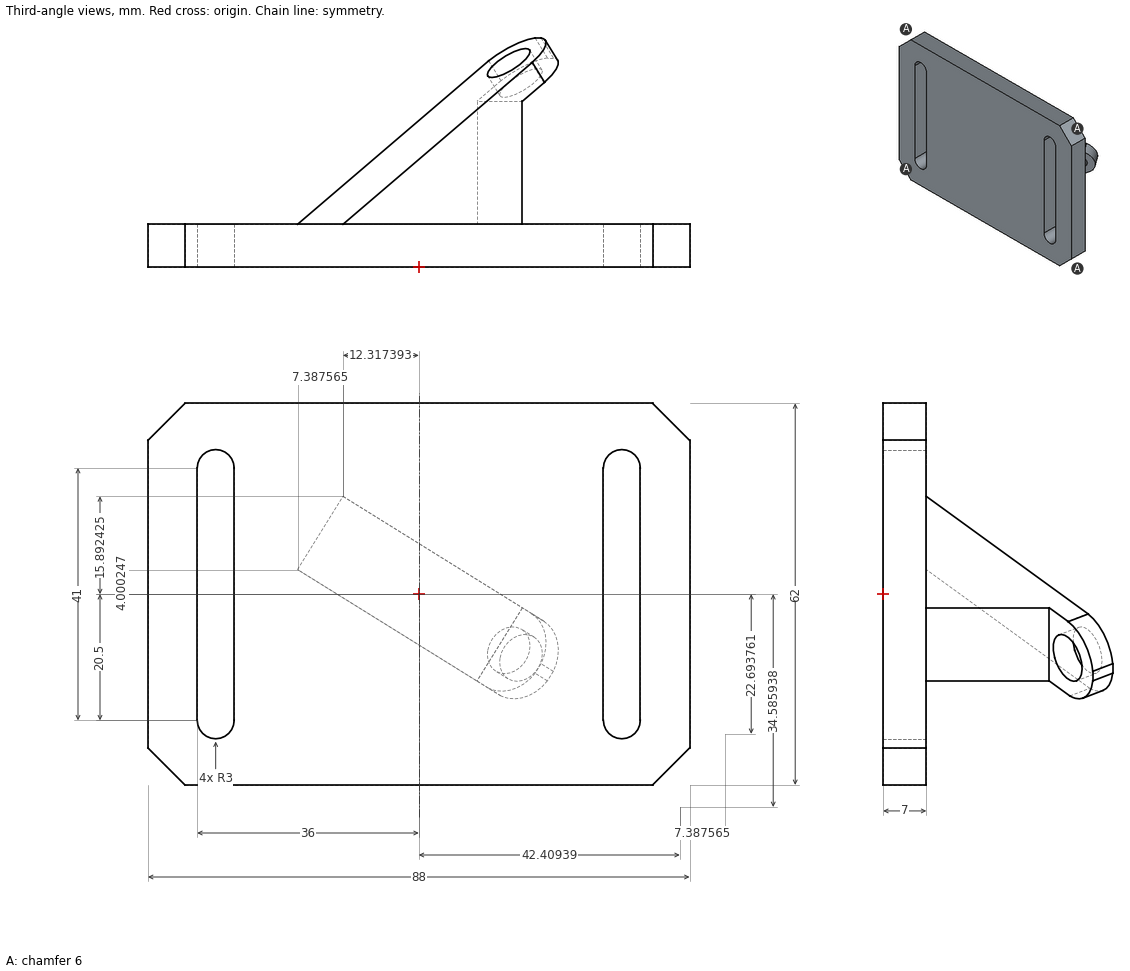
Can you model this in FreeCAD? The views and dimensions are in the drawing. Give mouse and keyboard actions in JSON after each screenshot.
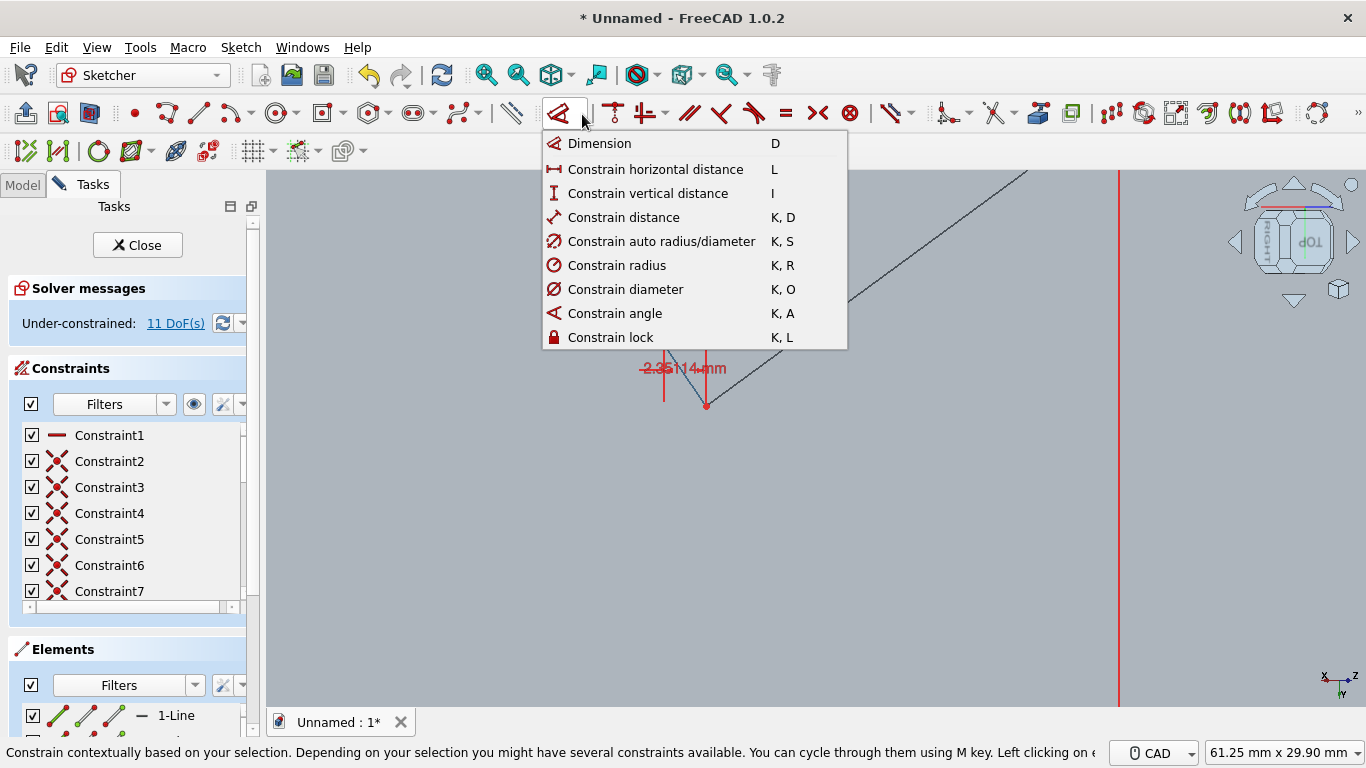
{"action": "left_click", "coordinate": [695, 193]}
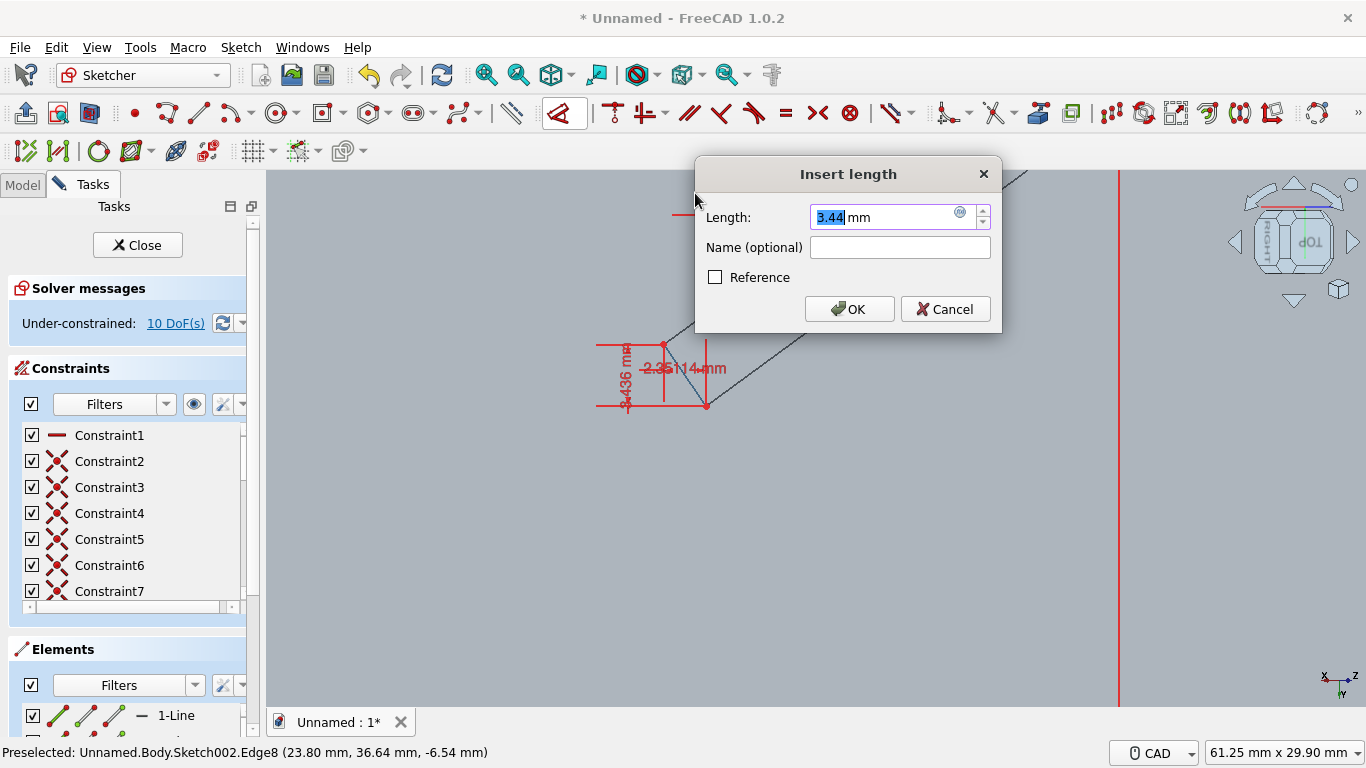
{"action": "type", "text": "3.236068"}
{"action": "key", "text": "Return"}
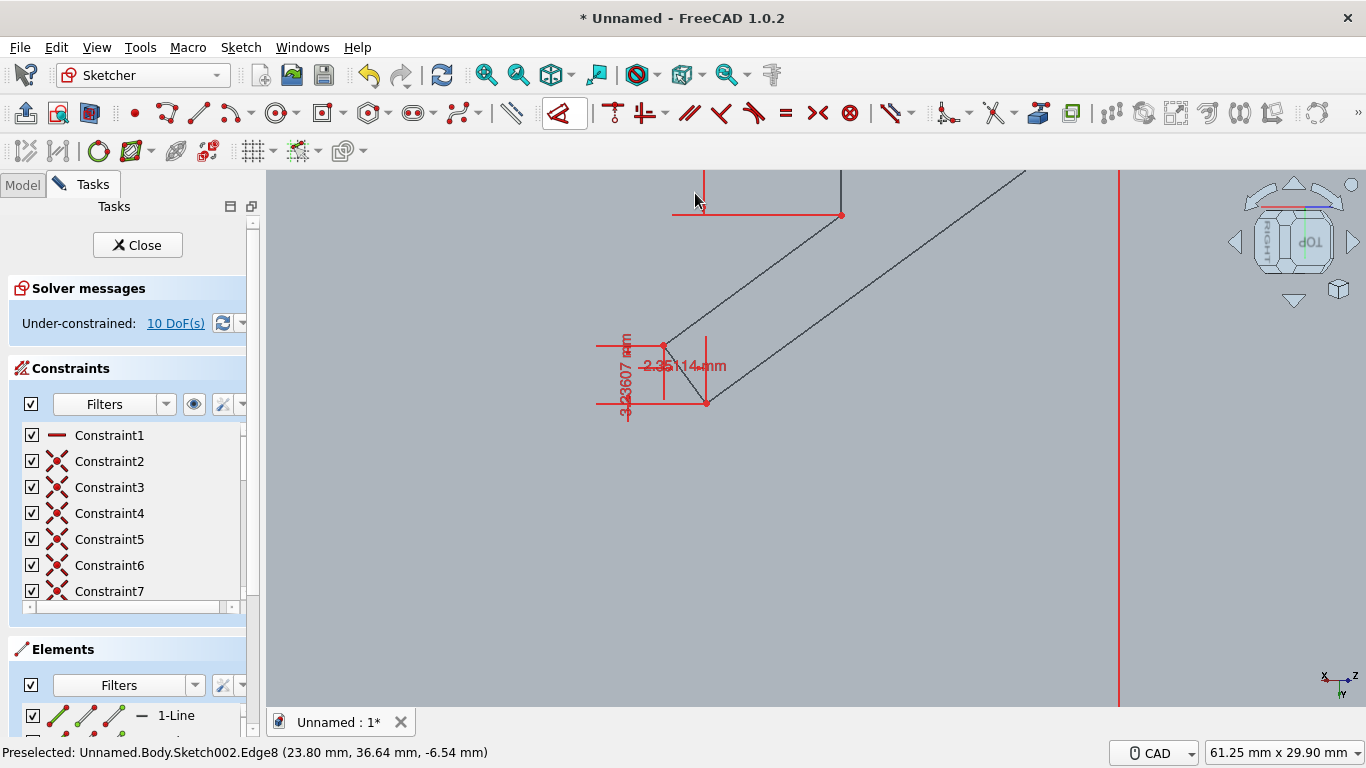
{"action": "scroll", "coordinate": [697, 389], "scroll_direction": "down", "scroll_amount": 9}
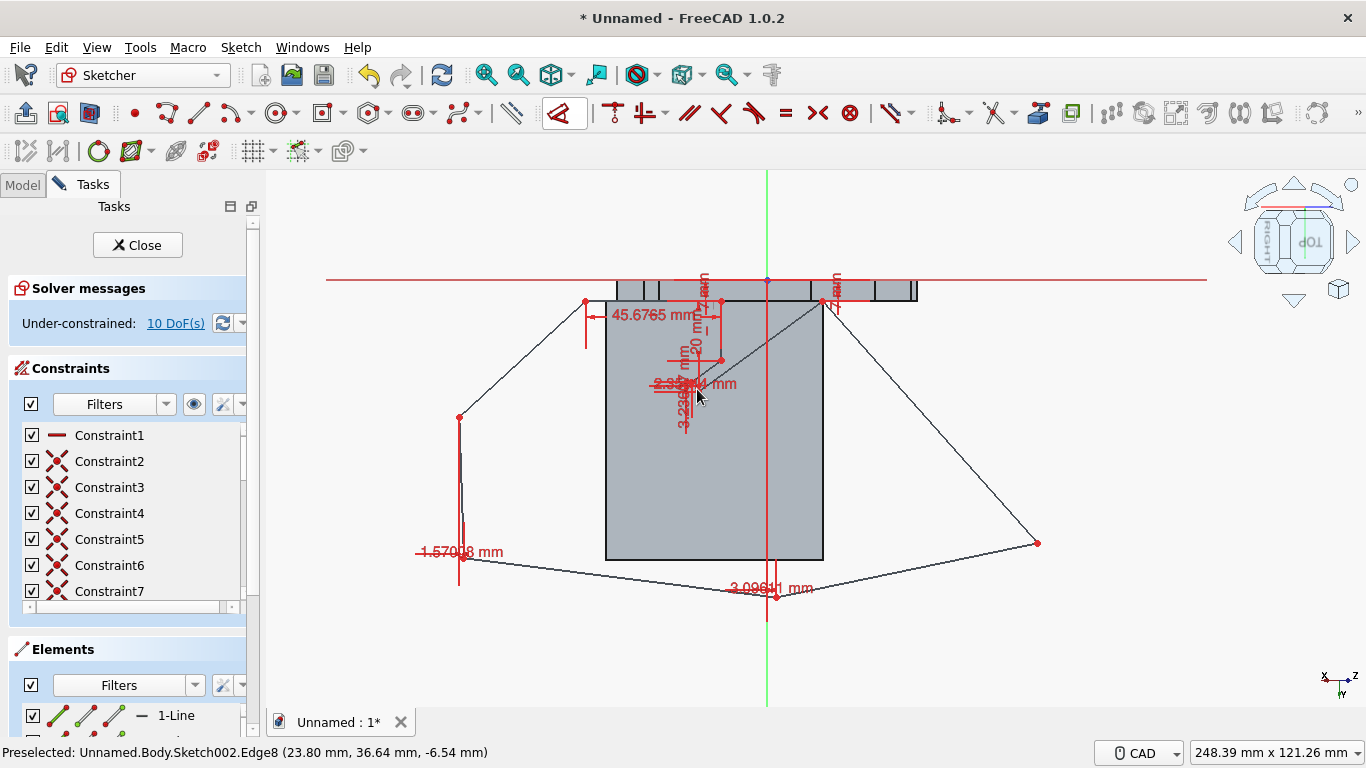
{"action": "scroll", "coordinate": [701, 376], "scroll_direction": "up", "scroll_amount": 2}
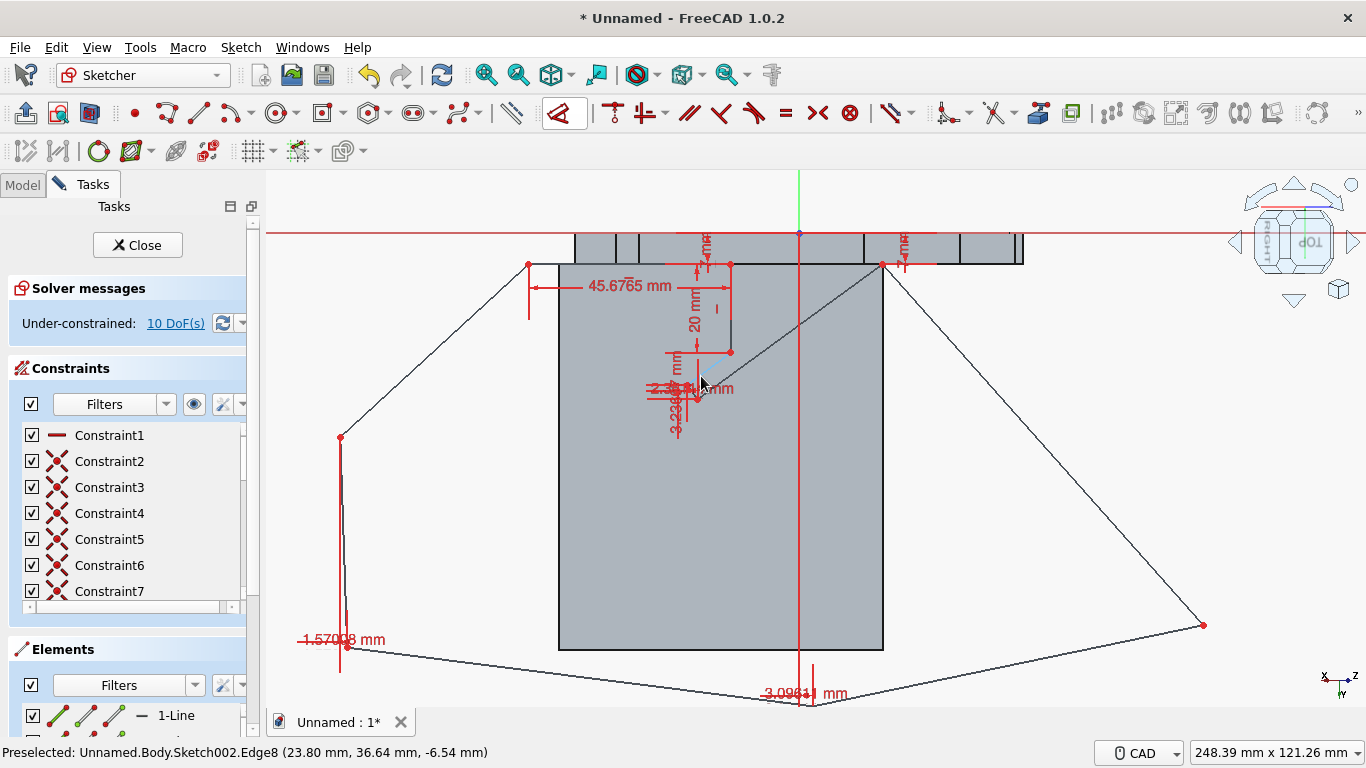
{"action": "left_click", "coordinate": [700, 375]}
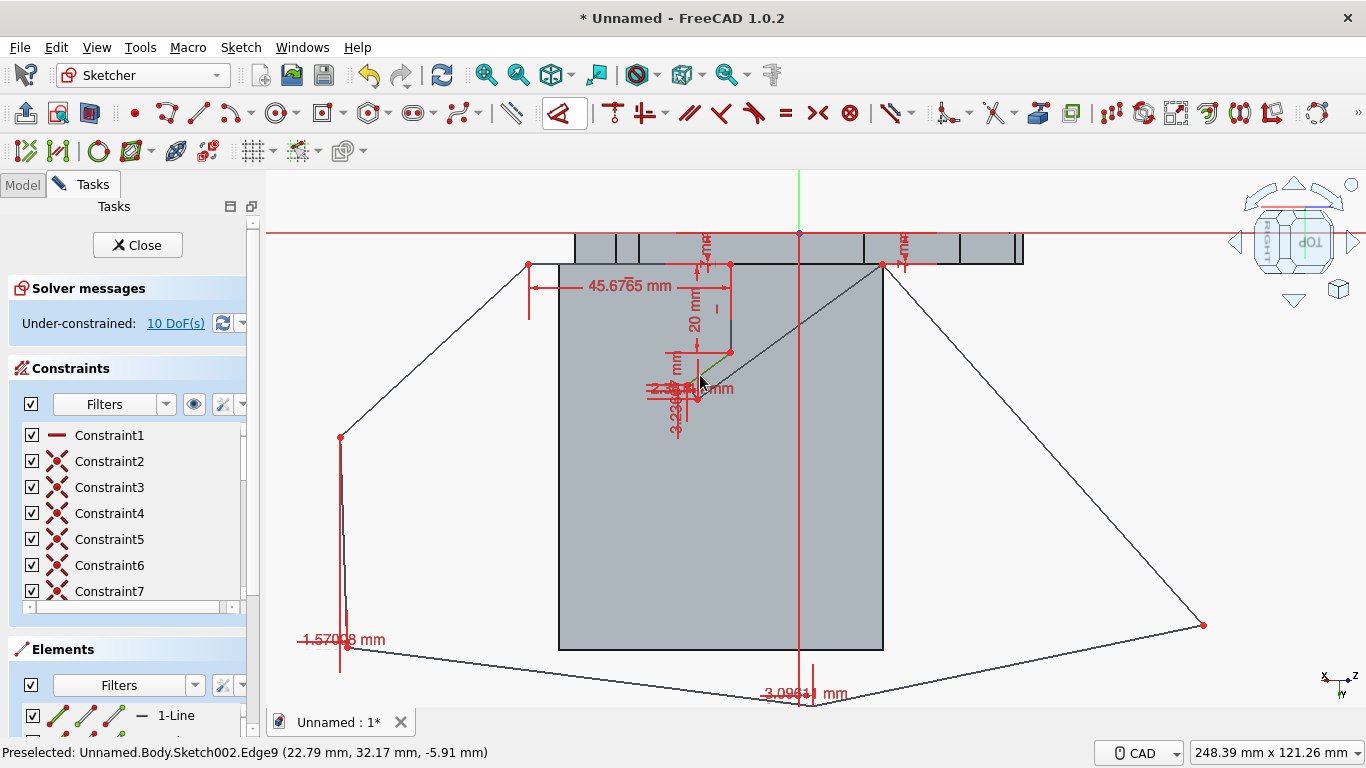
{"action": "left_click", "coordinate": [582, 114]}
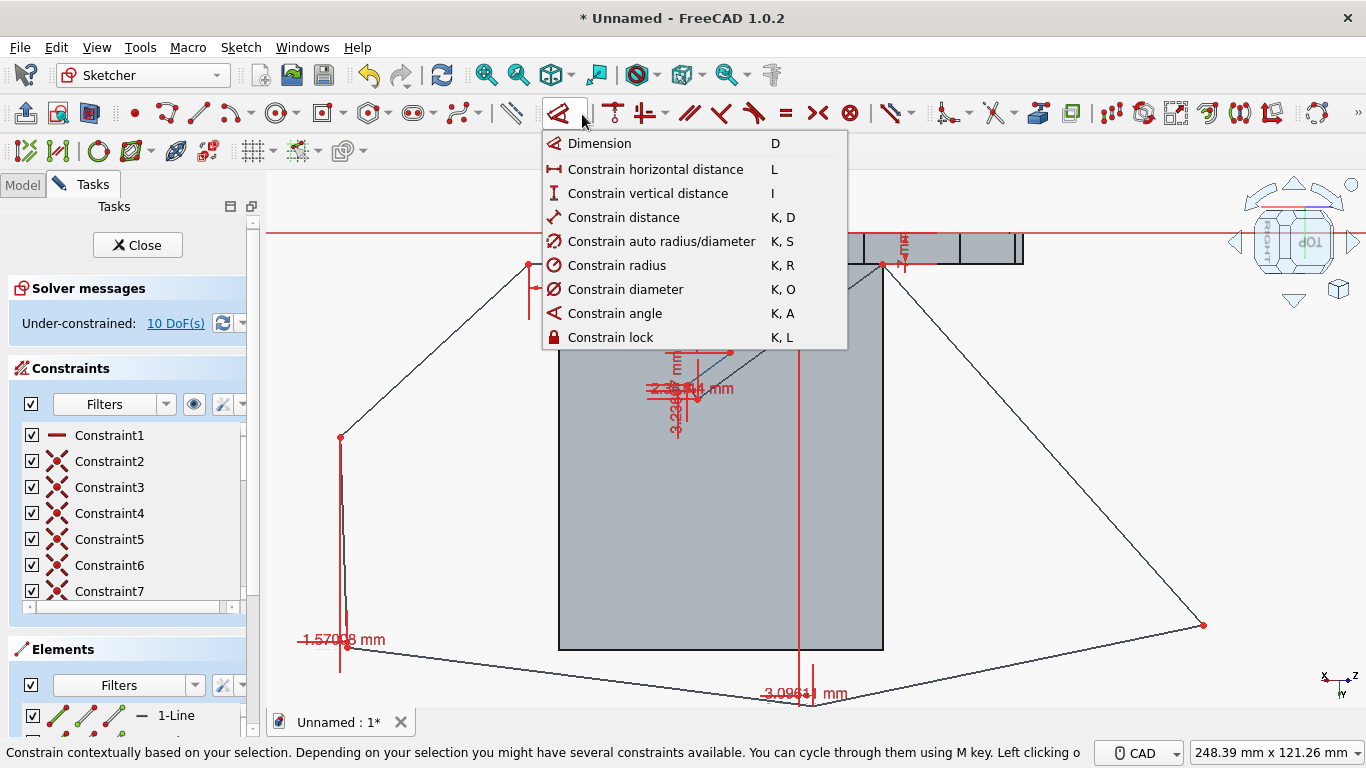
{"action": "left_click", "coordinate": [695, 169]}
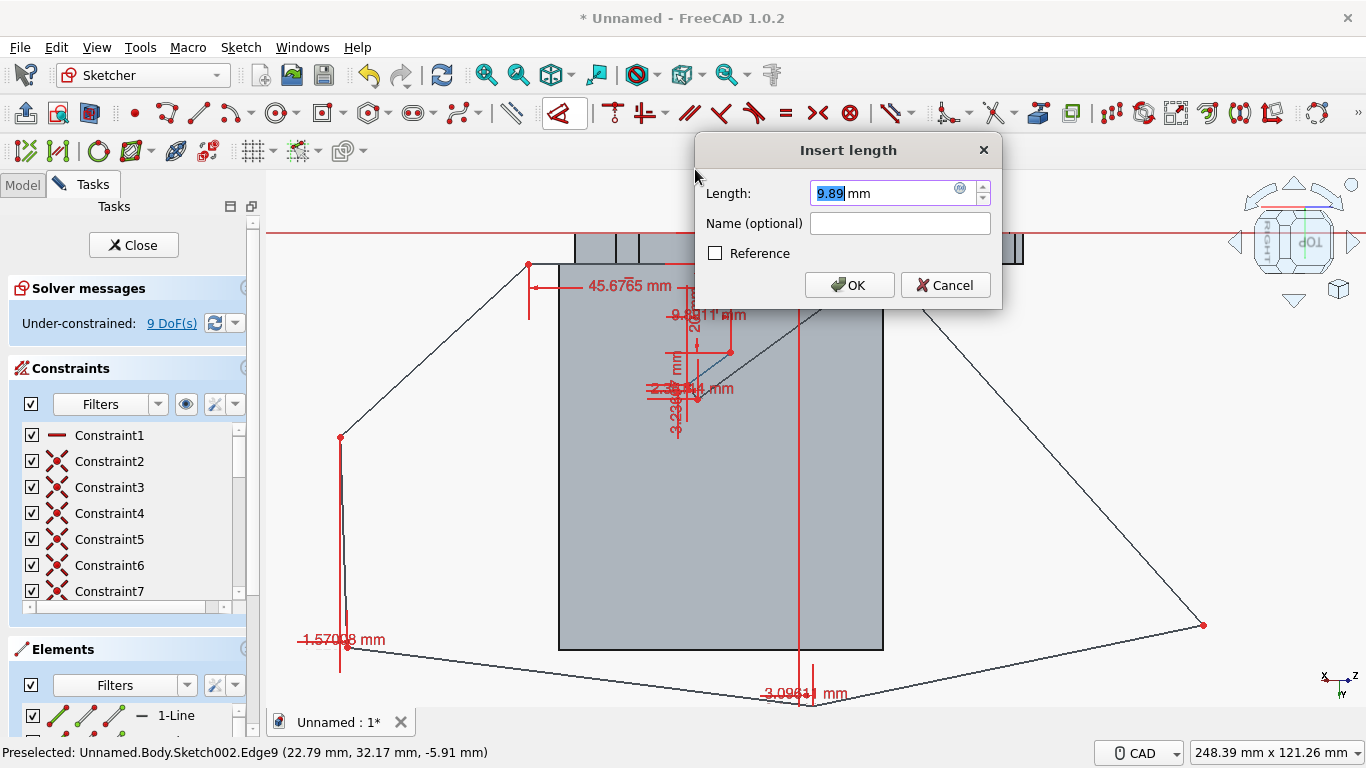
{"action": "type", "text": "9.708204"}
{"action": "key", "text": "Return"}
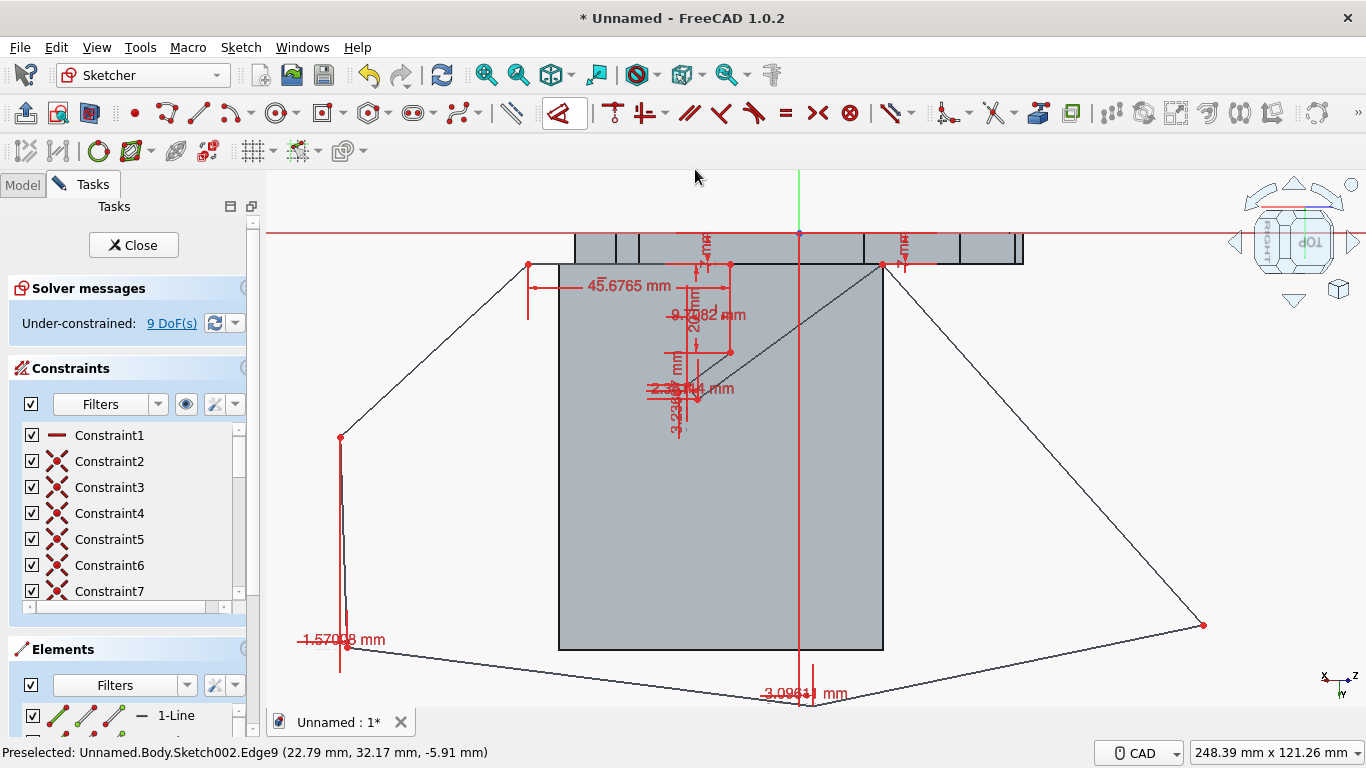
{"action": "scroll", "coordinate": [700, 375], "scroll_direction": "up", "scroll_amount": 2}